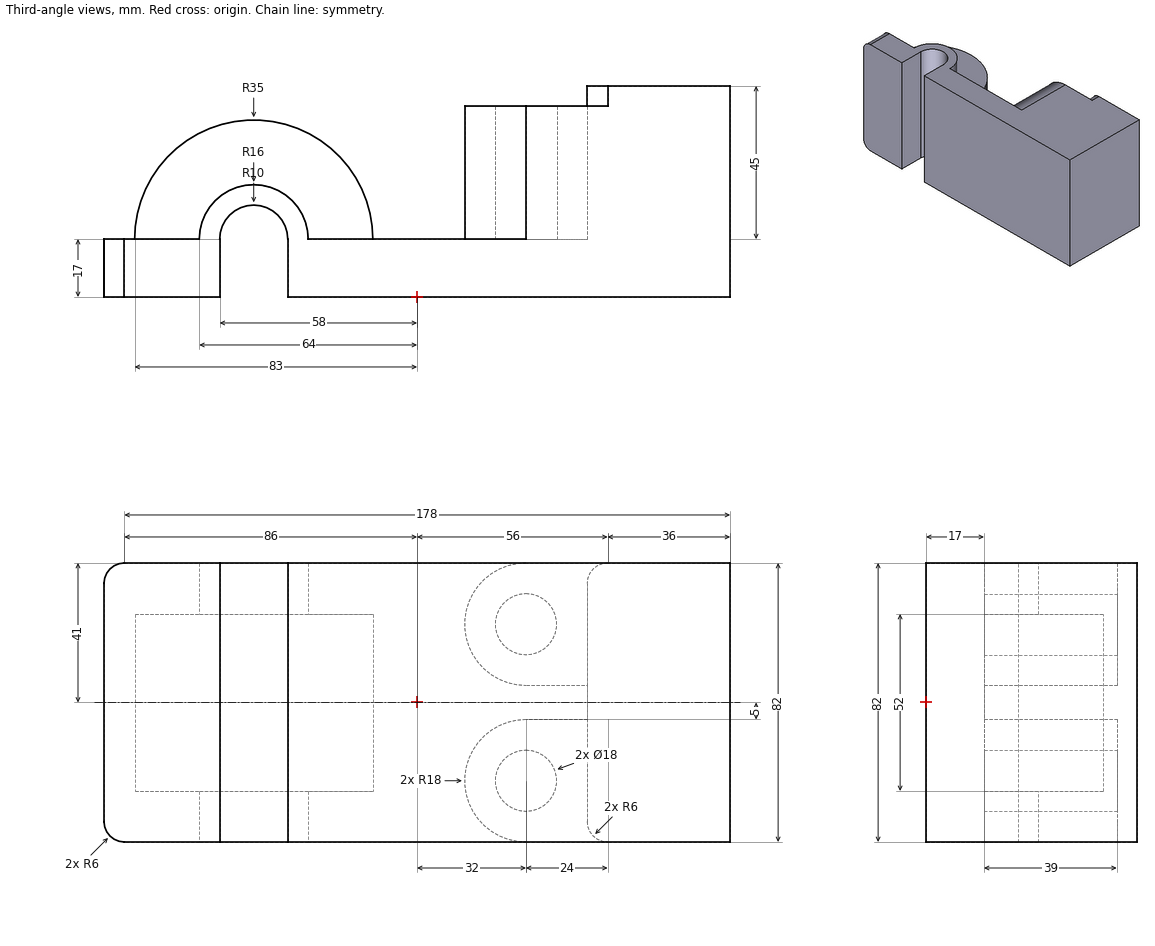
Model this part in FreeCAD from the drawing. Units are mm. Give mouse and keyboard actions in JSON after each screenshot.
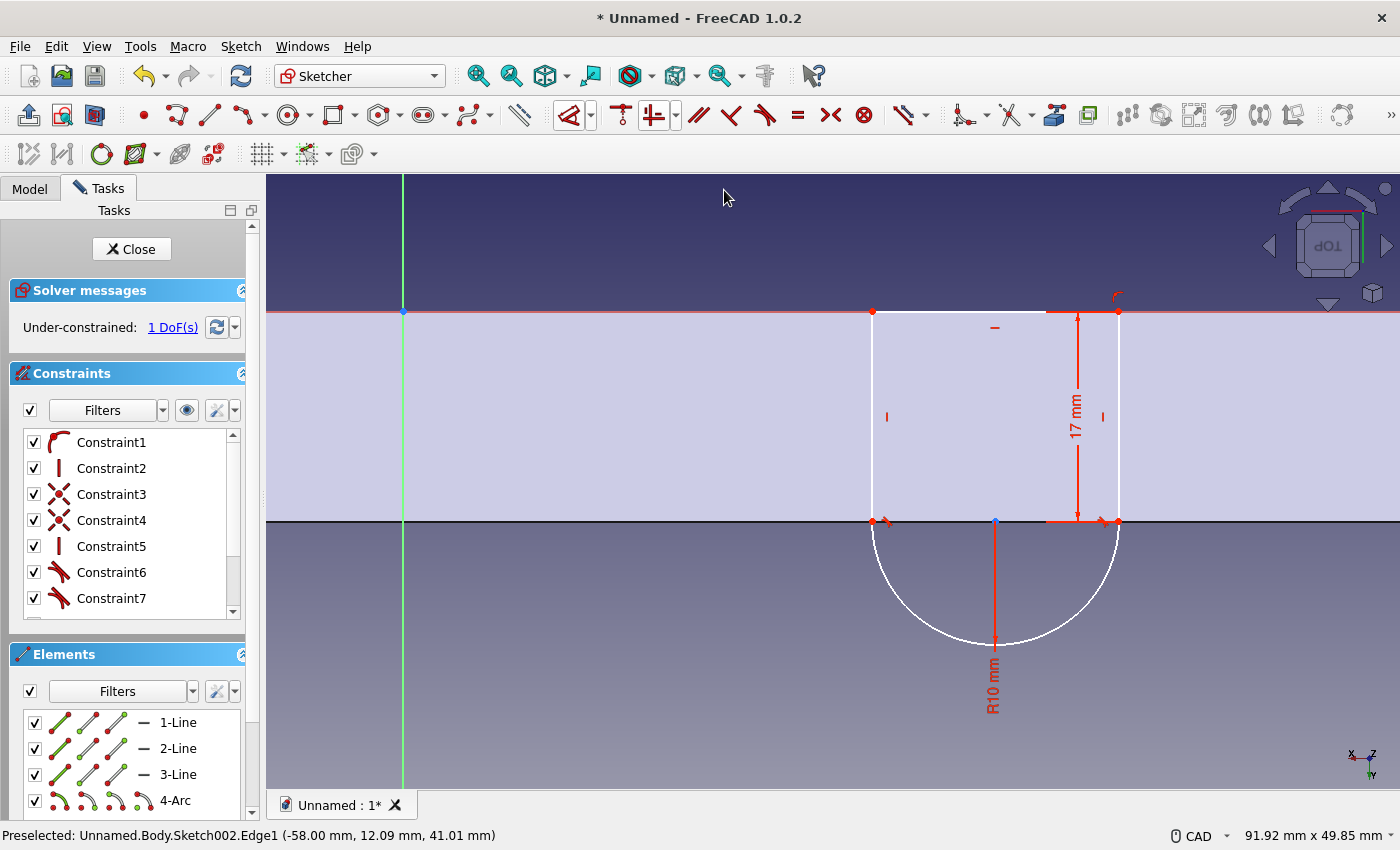
{"action": "left_click", "coordinate": [1119, 522]}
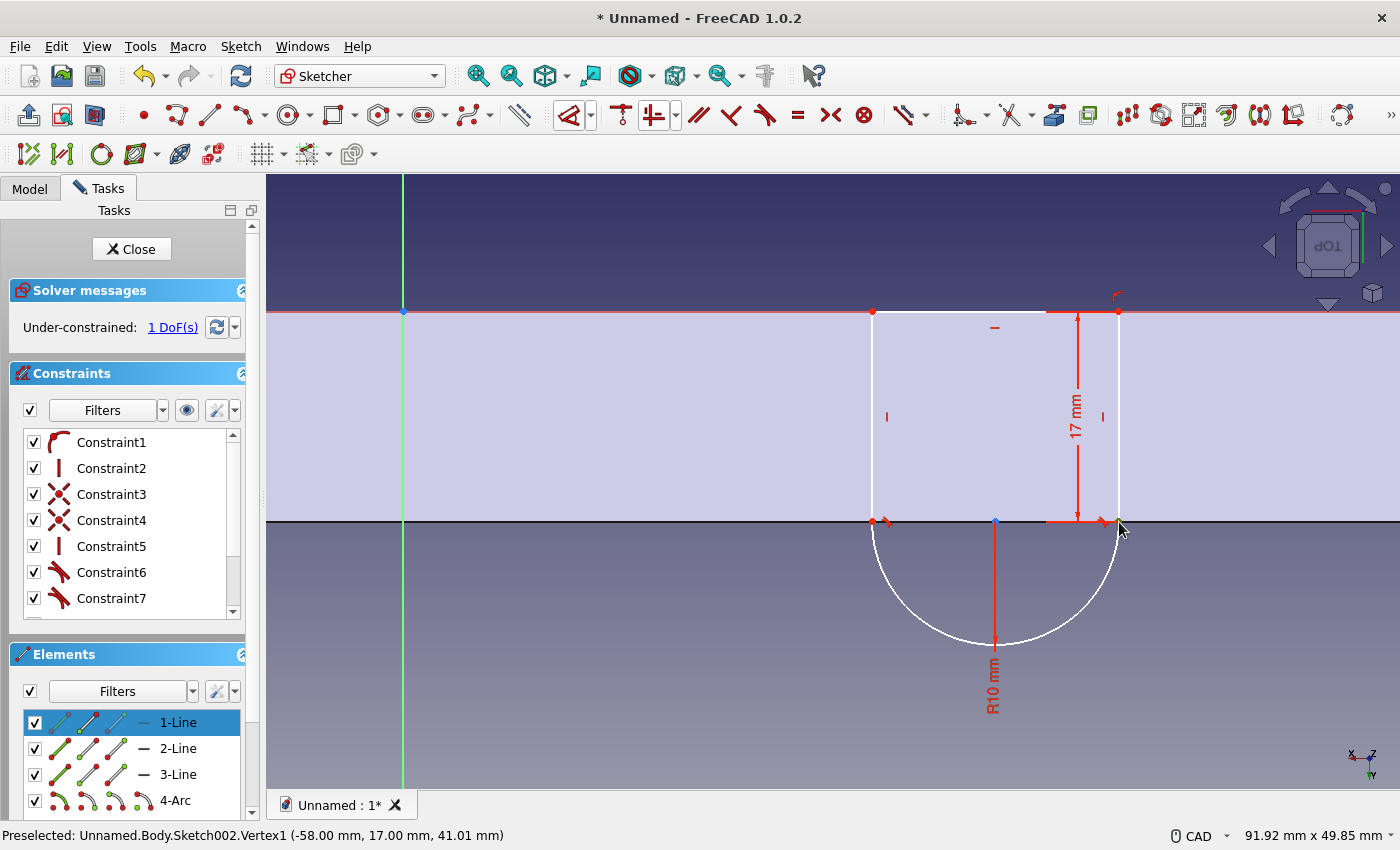
{"action": "key", "text": "l"}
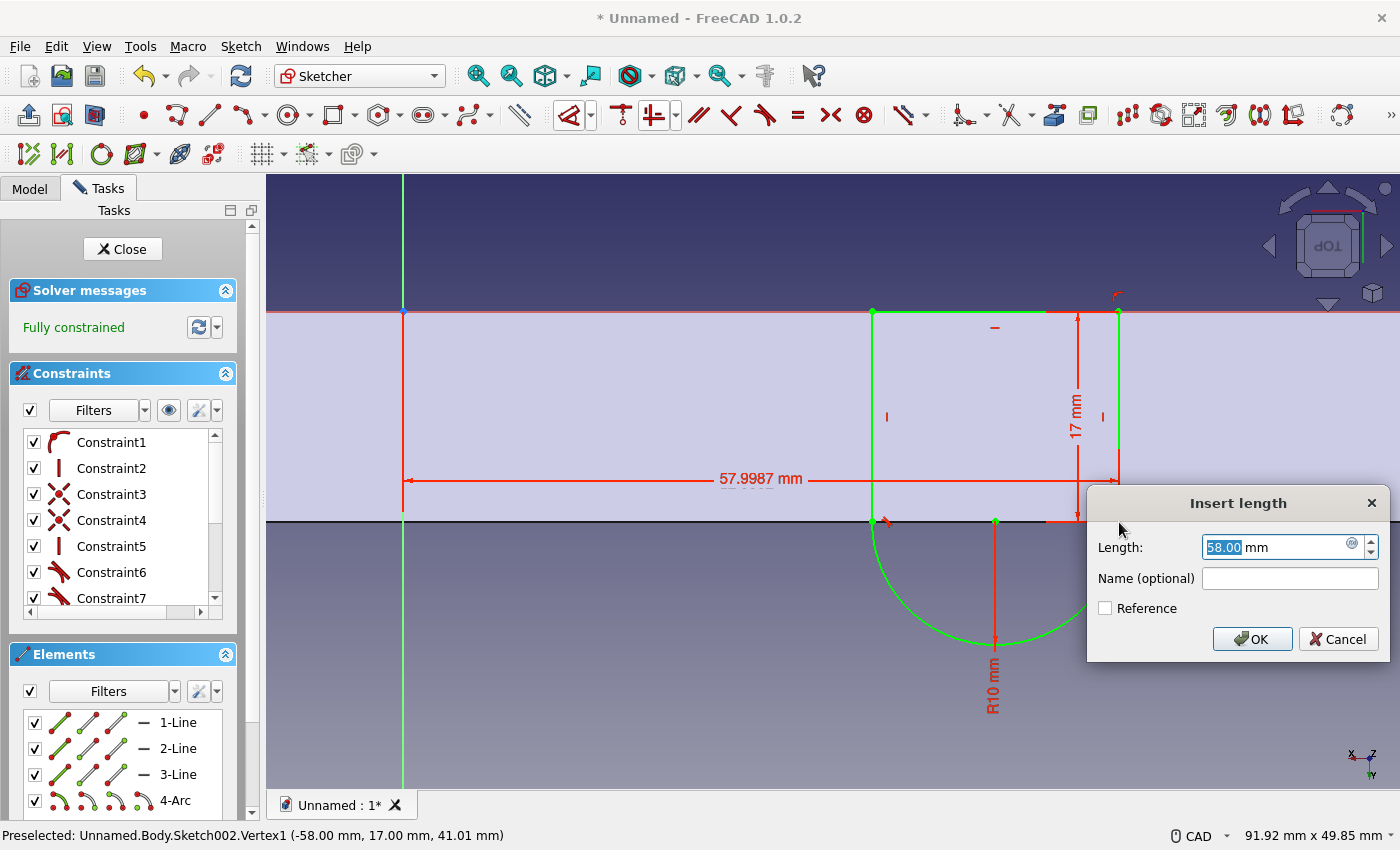
{"action": "type", "text": "58"}
{"action": "key", "text": "Return"}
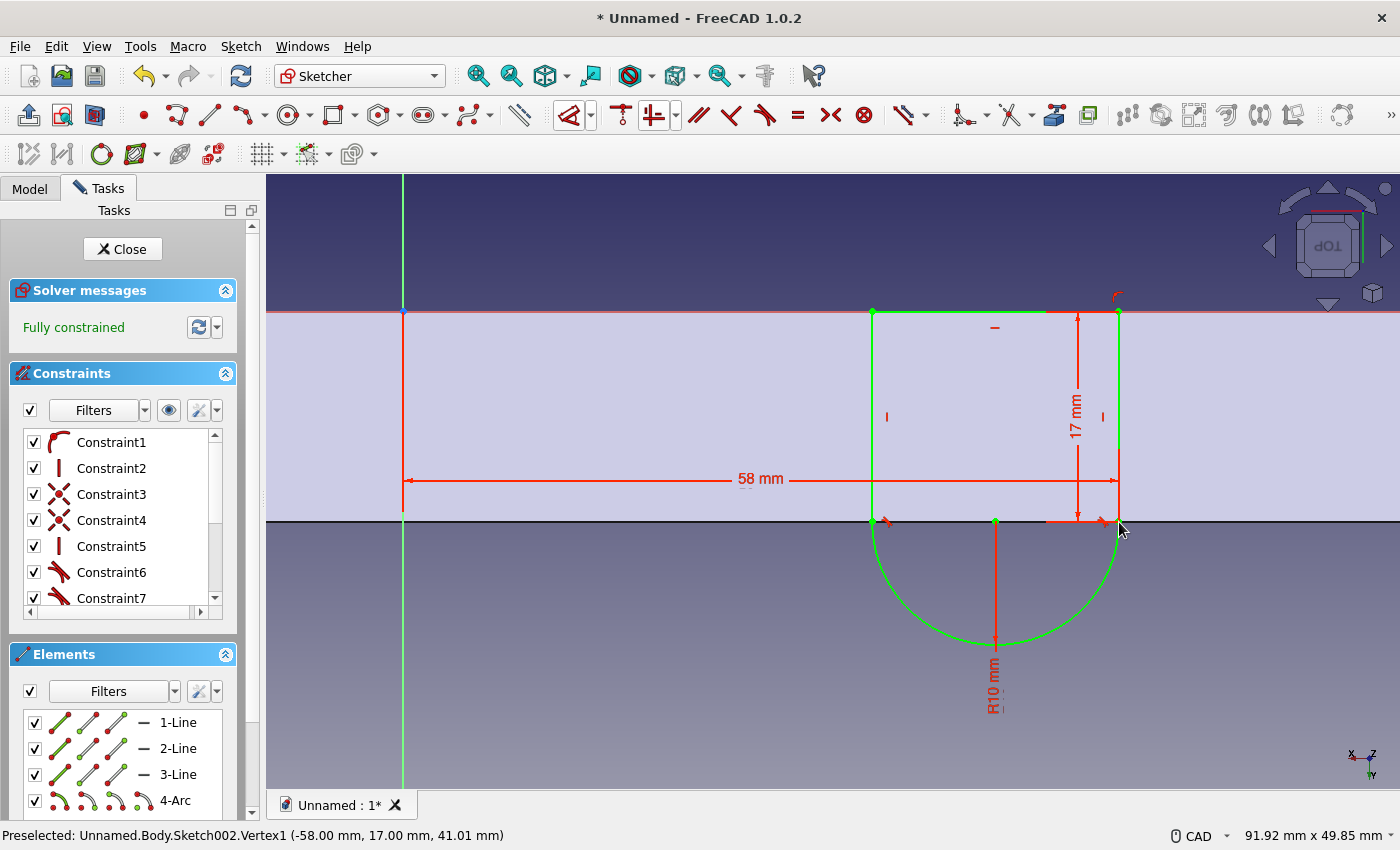
{"action": "left_click", "coordinate": [123, 249]}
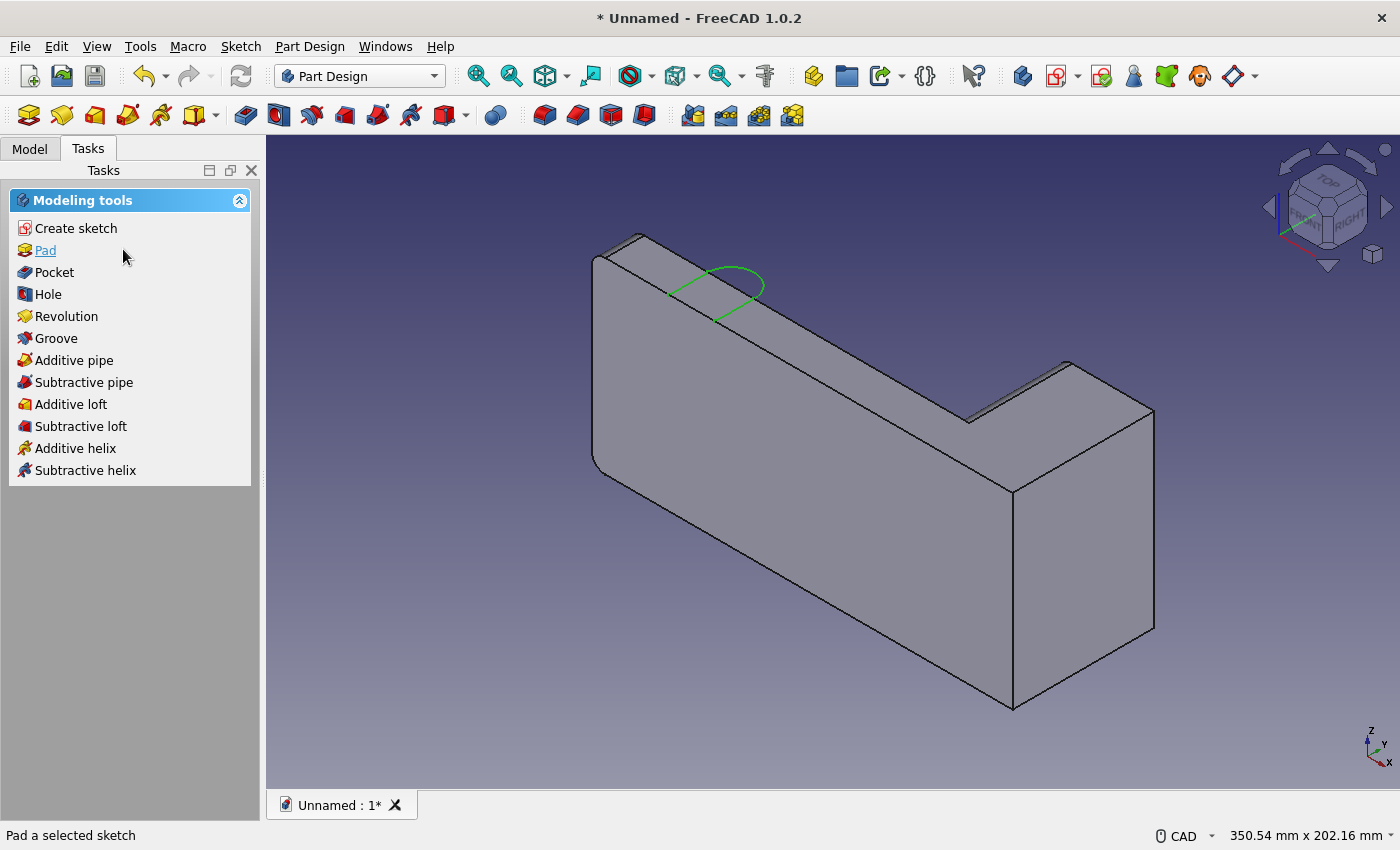
{"action": "left_click", "coordinate": [29, 116]}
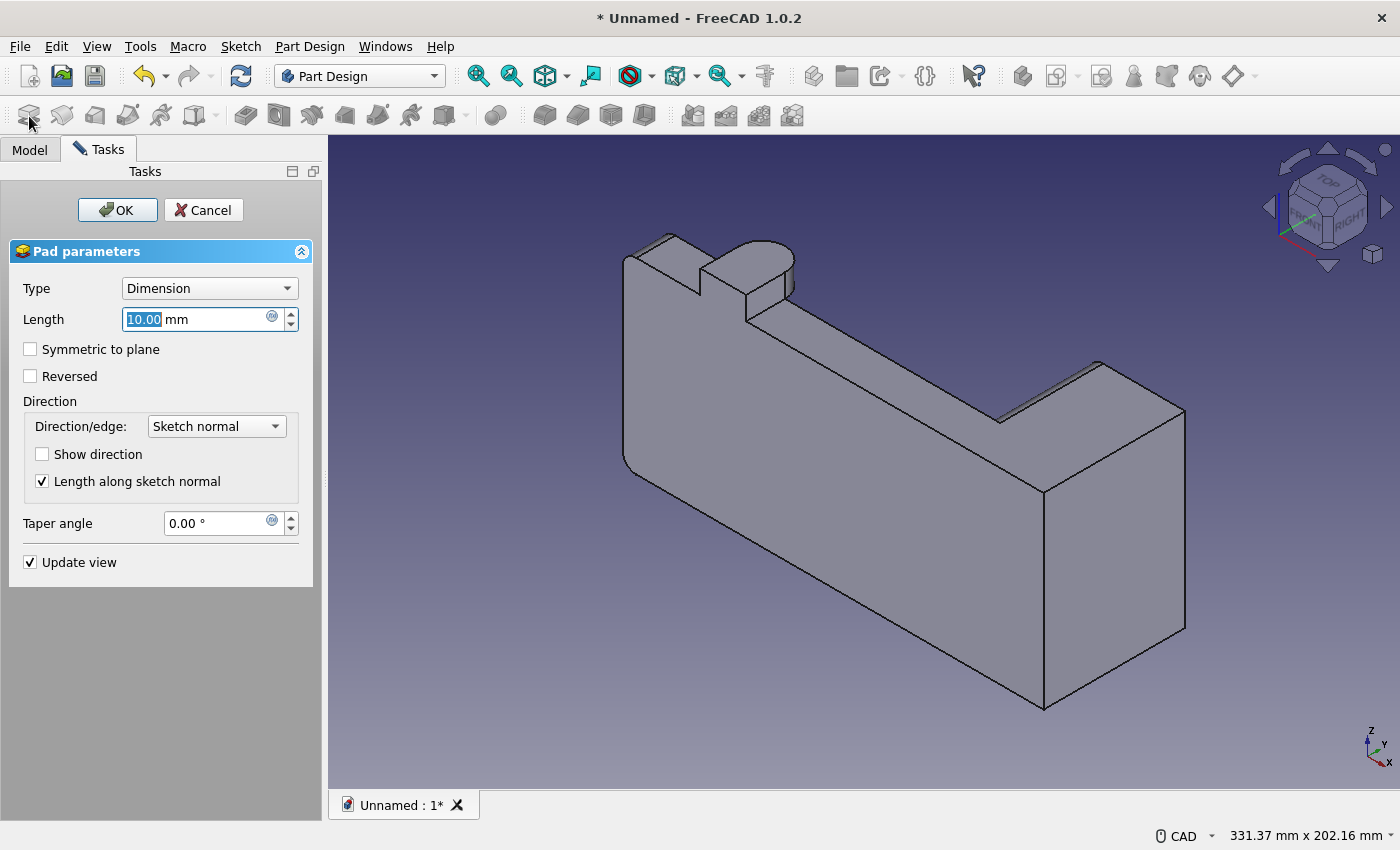
{"action": "type", "text": "82"}
{"action": "key", "text": "Tab"}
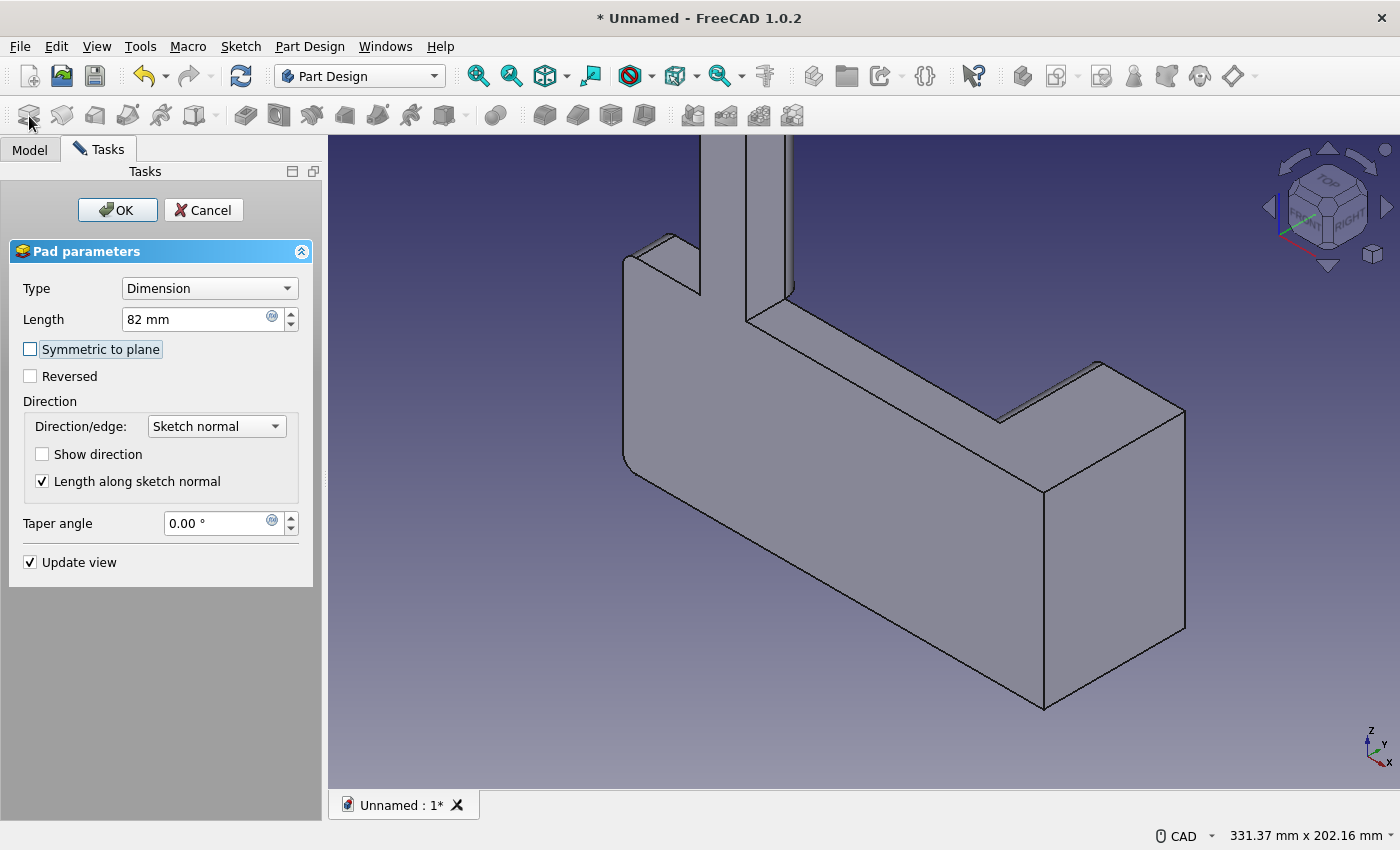
{"action": "left_click", "coordinate": [31, 376]}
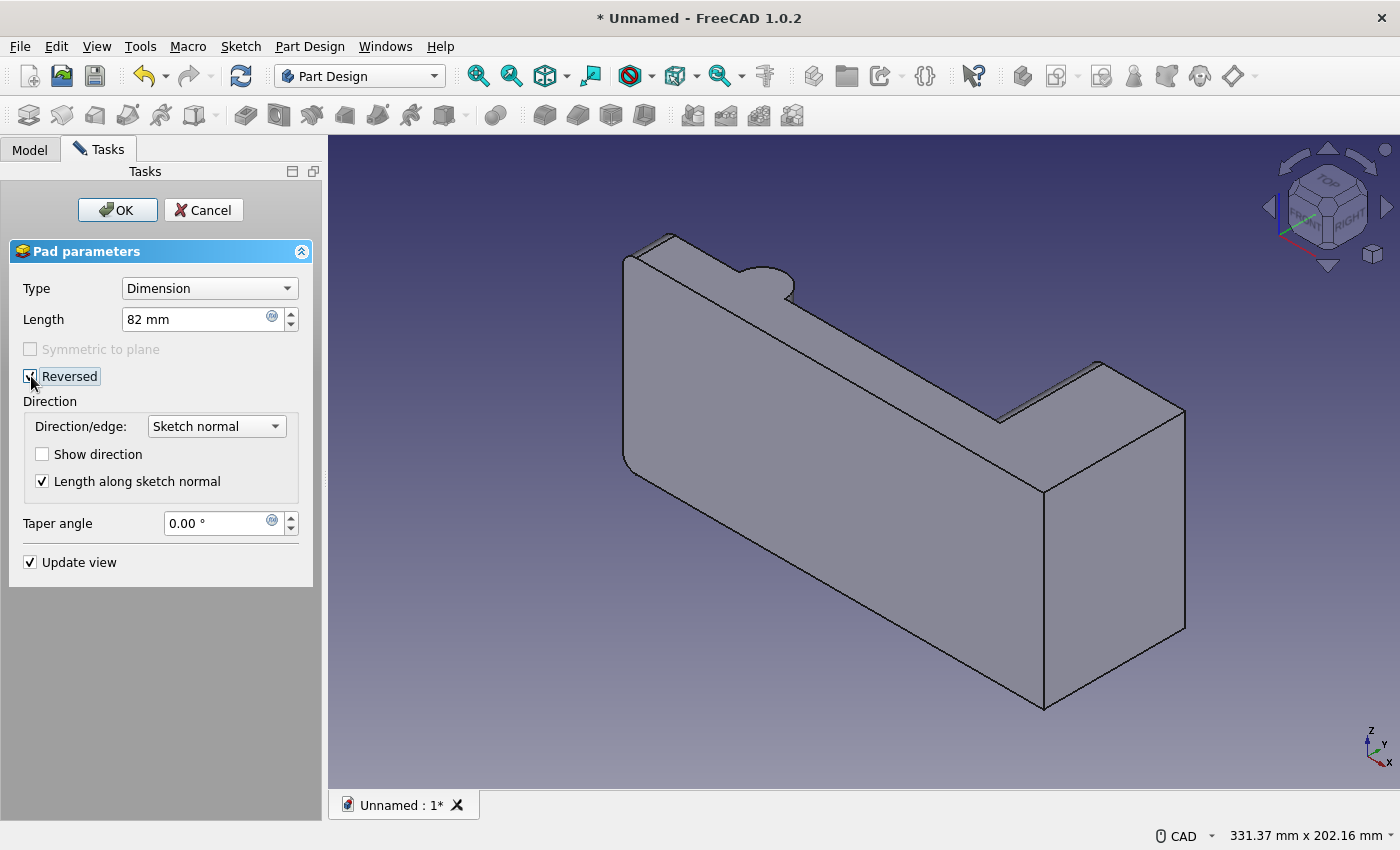
{"action": "left_click", "coordinate": [118, 210]}